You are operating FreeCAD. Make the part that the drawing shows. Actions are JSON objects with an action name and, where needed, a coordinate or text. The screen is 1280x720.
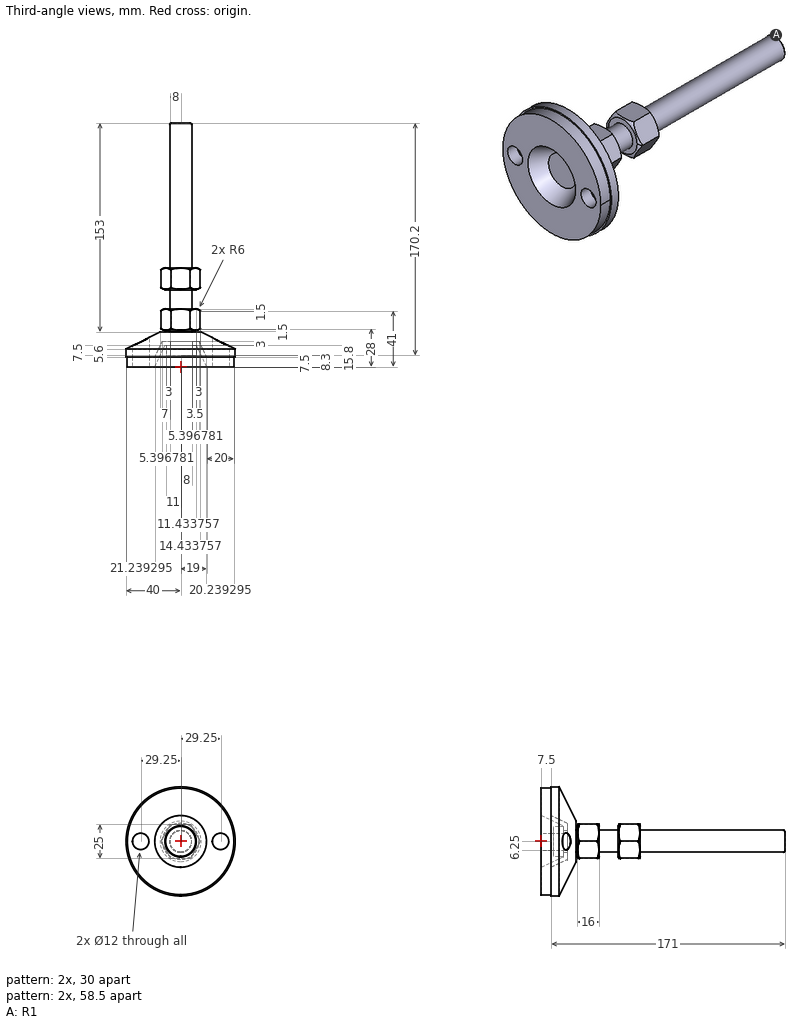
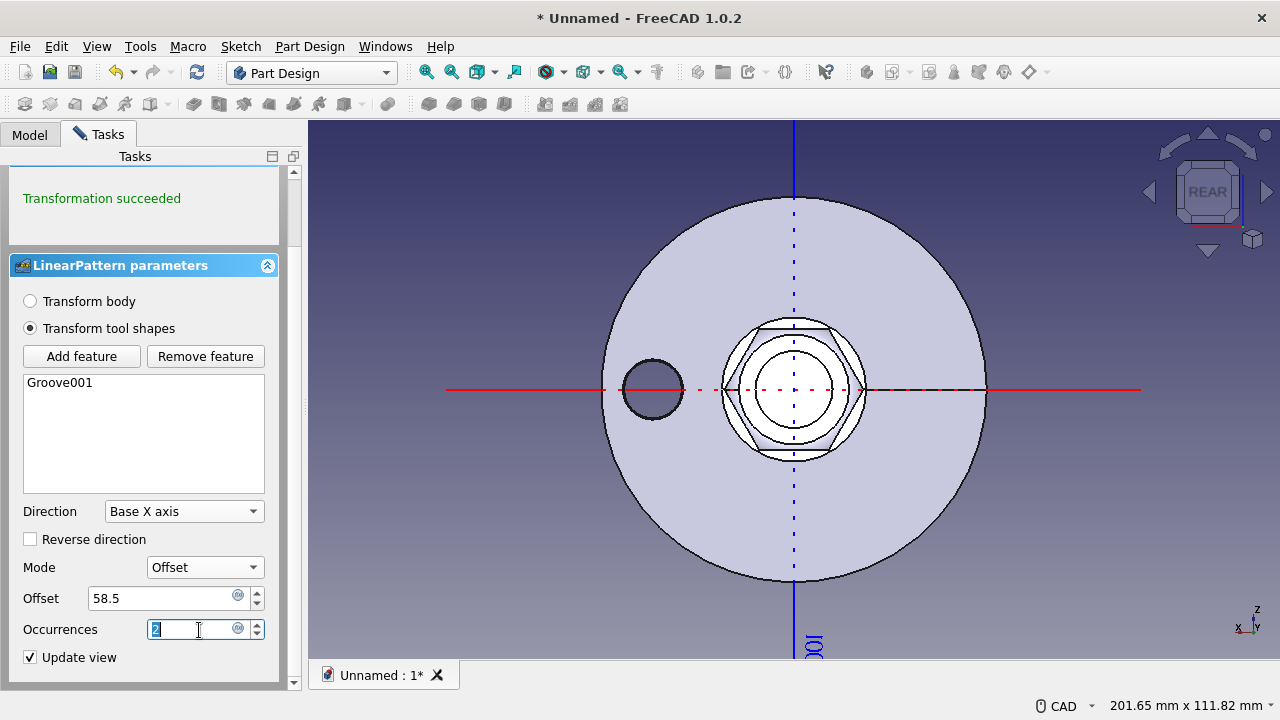
{"action": "type", "text": "2"}
{"action": "key", "text": "Tab"}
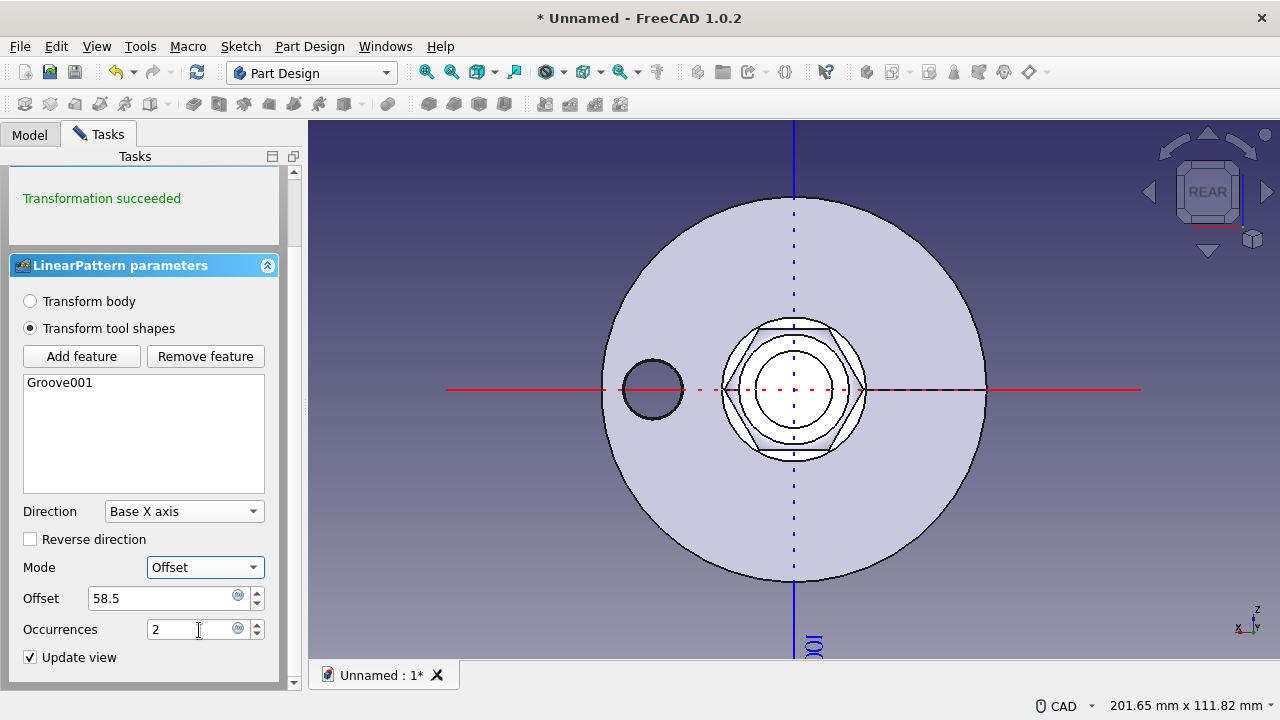
{"action": "left_click", "coordinate": [31, 539]}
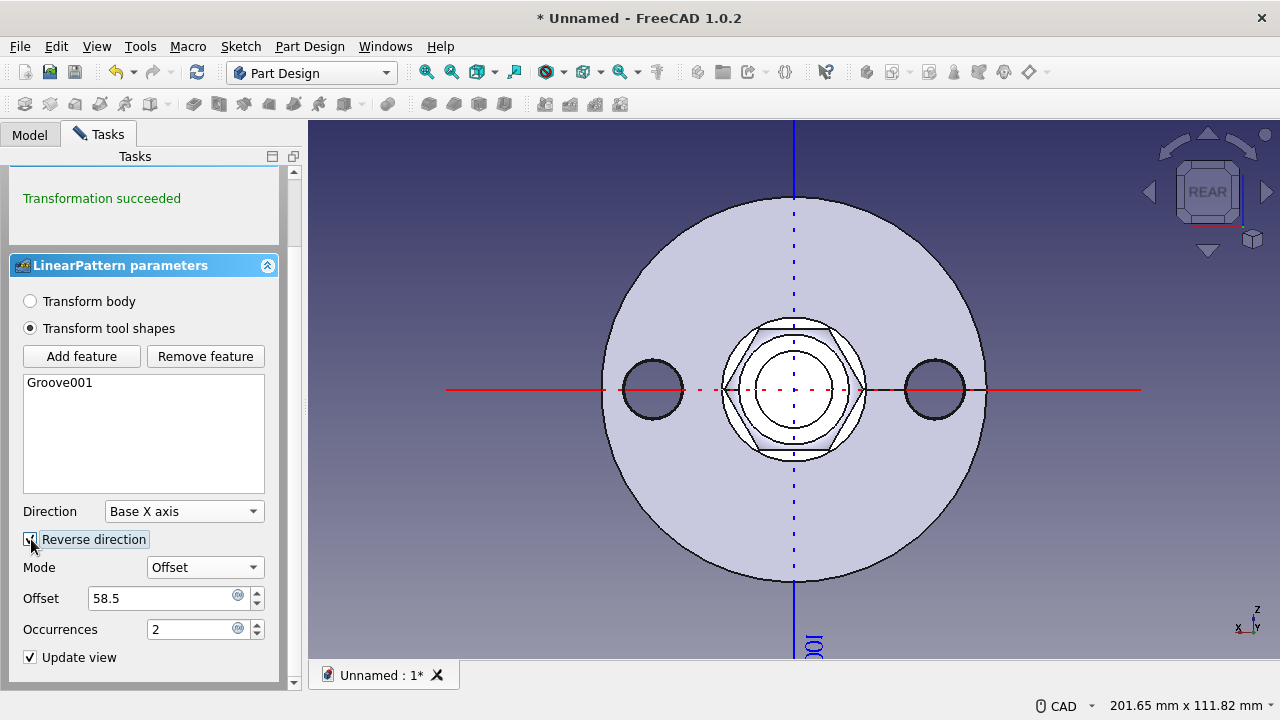
{"action": "scroll", "coordinate": [294, 428], "scroll_direction": "up", "scroll_amount": 3}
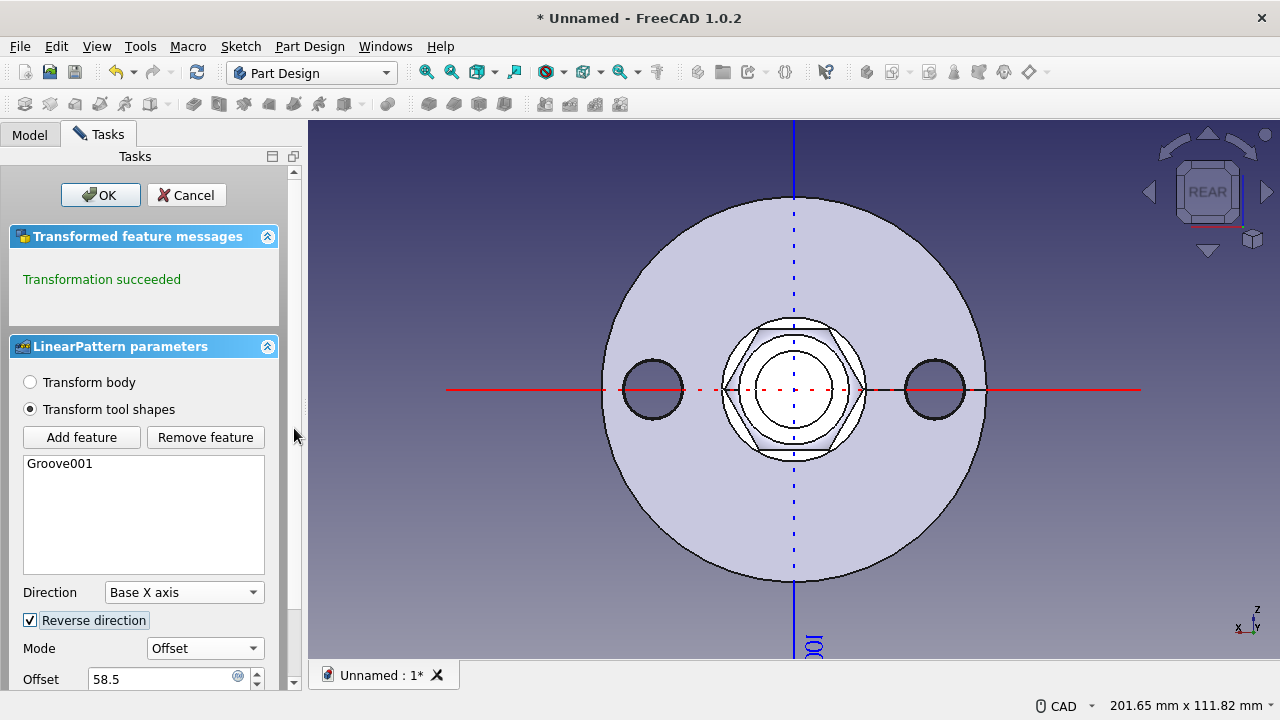
{"action": "left_click", "coordinate": [101, 195]}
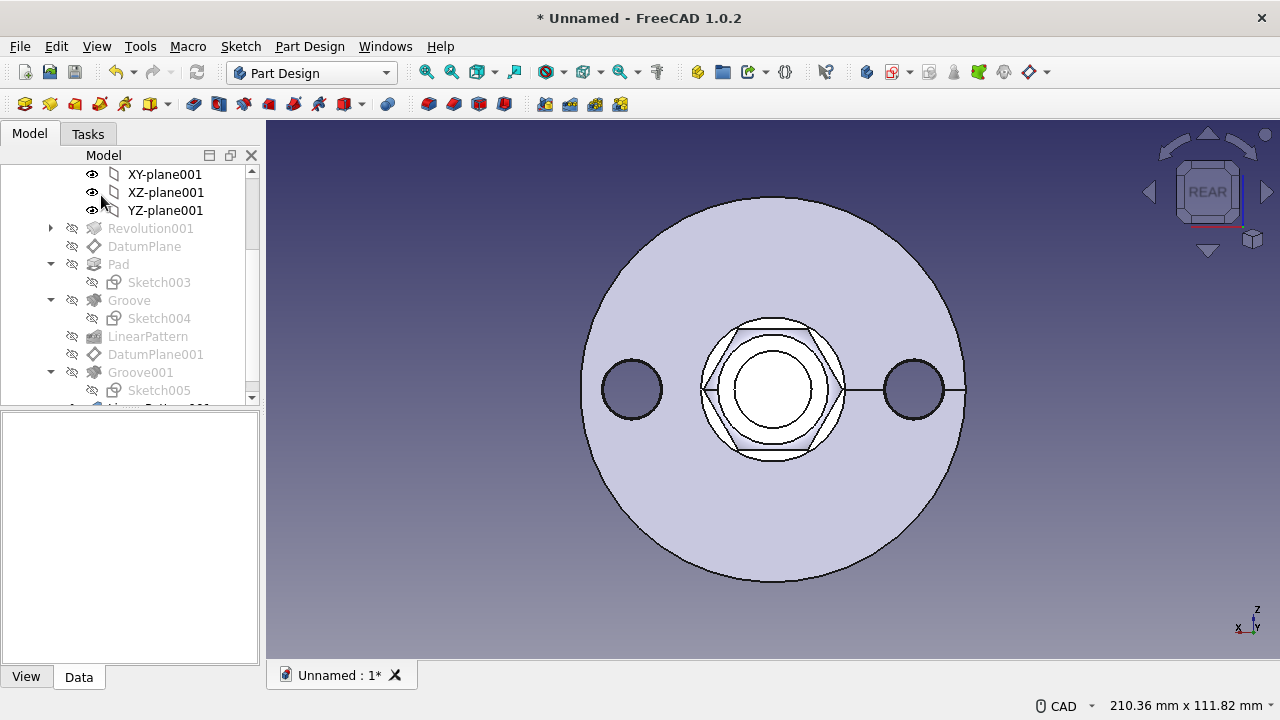
{"action": "left_click", "coordinate": [742, 366]}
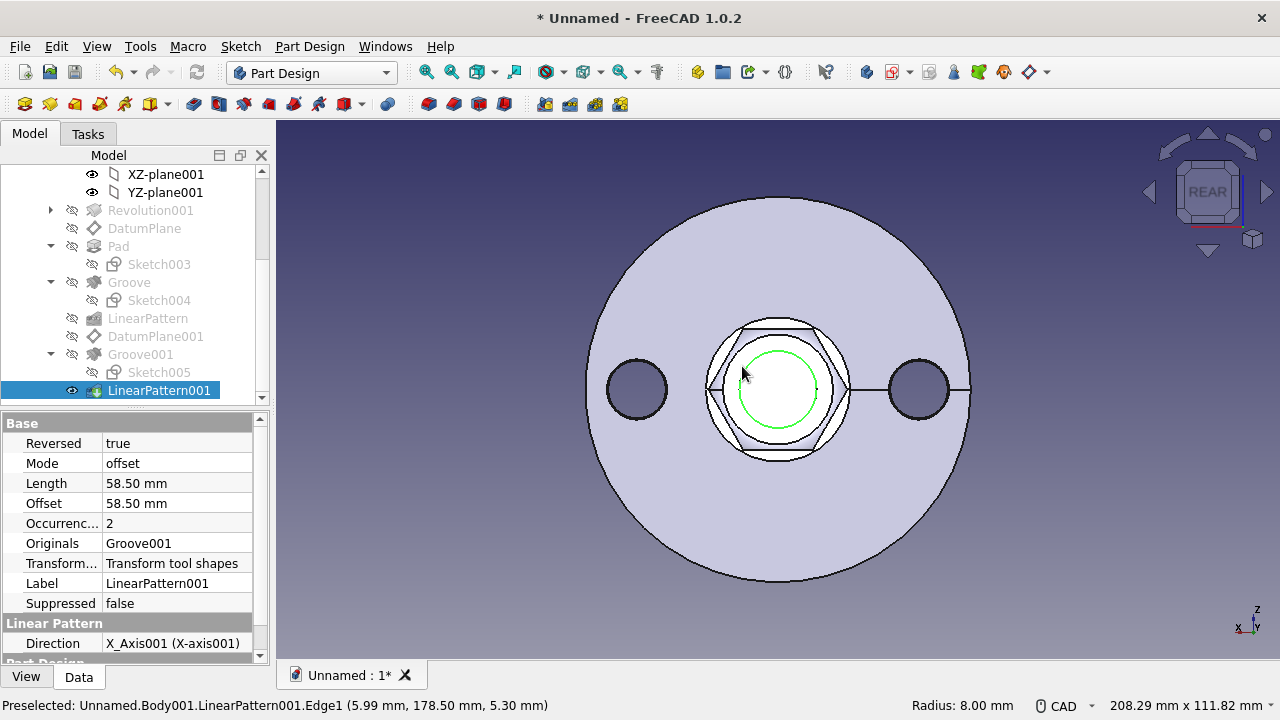
{"action": "left_click", "coordinate": [429, 104]}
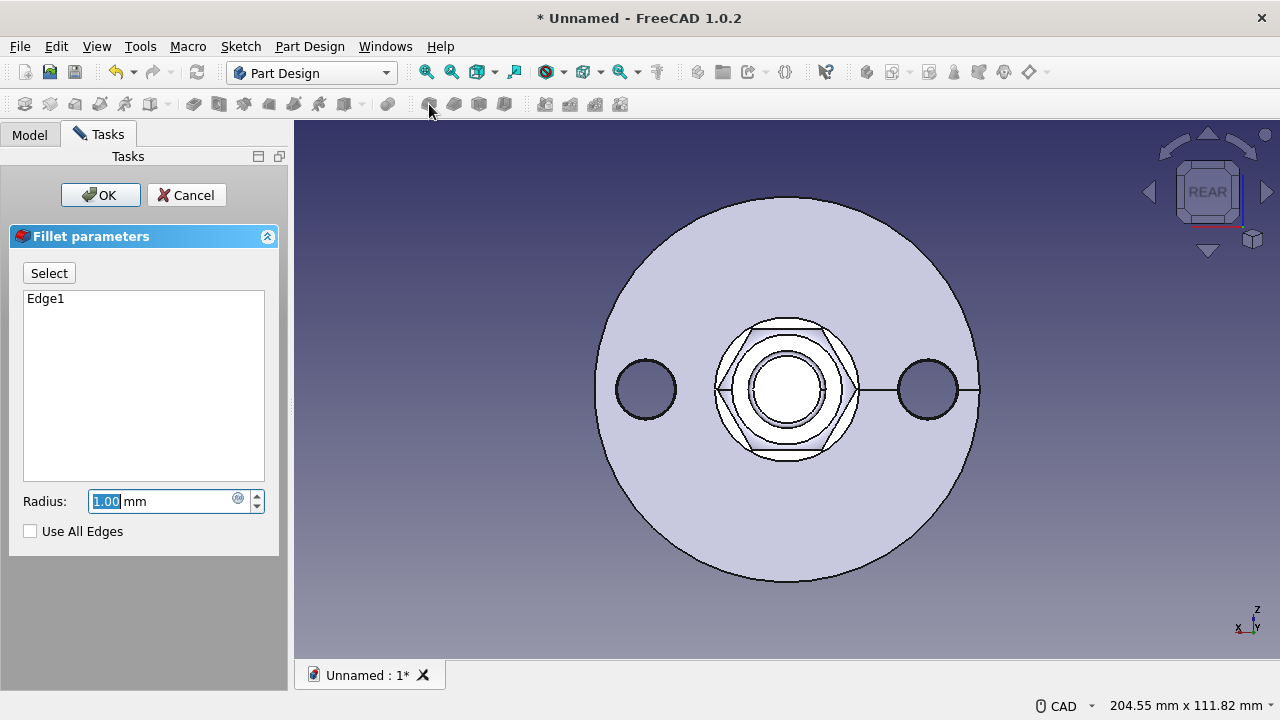
{"action": "type", "text": "1"}
{"action": "key", "text": "Tab"}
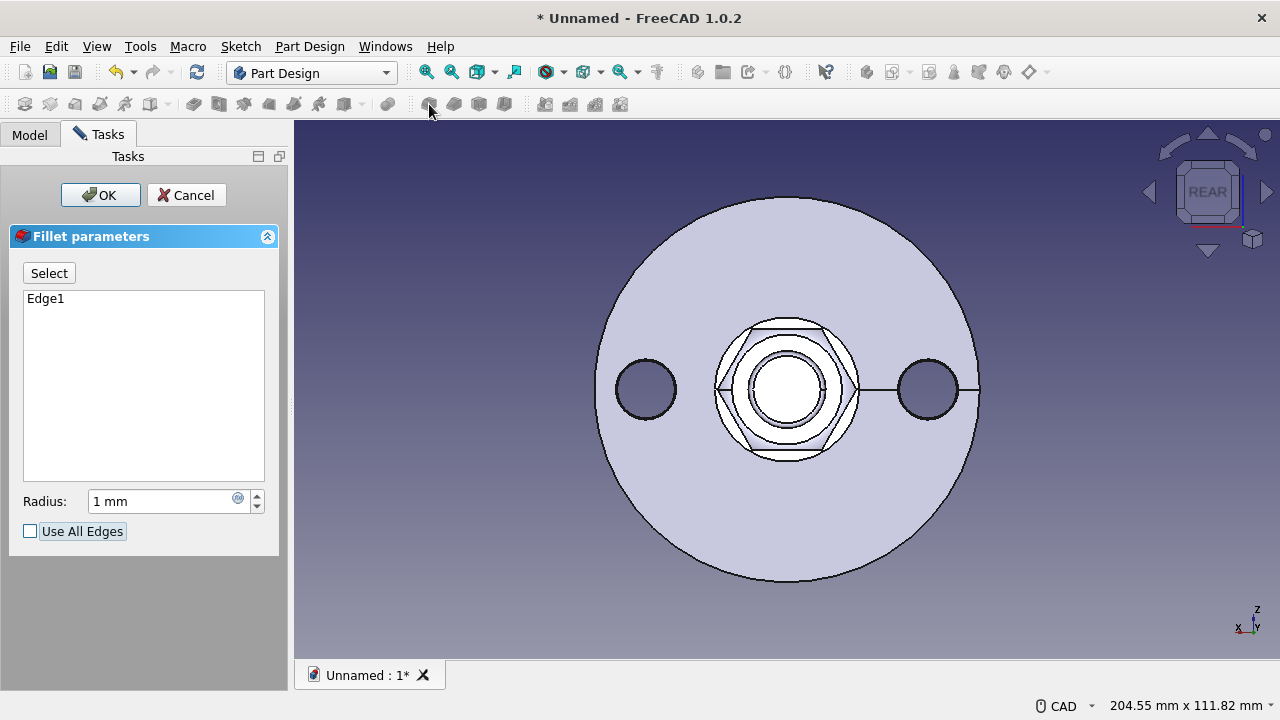
{"action": "left_click", "coordinate": [101, 195]}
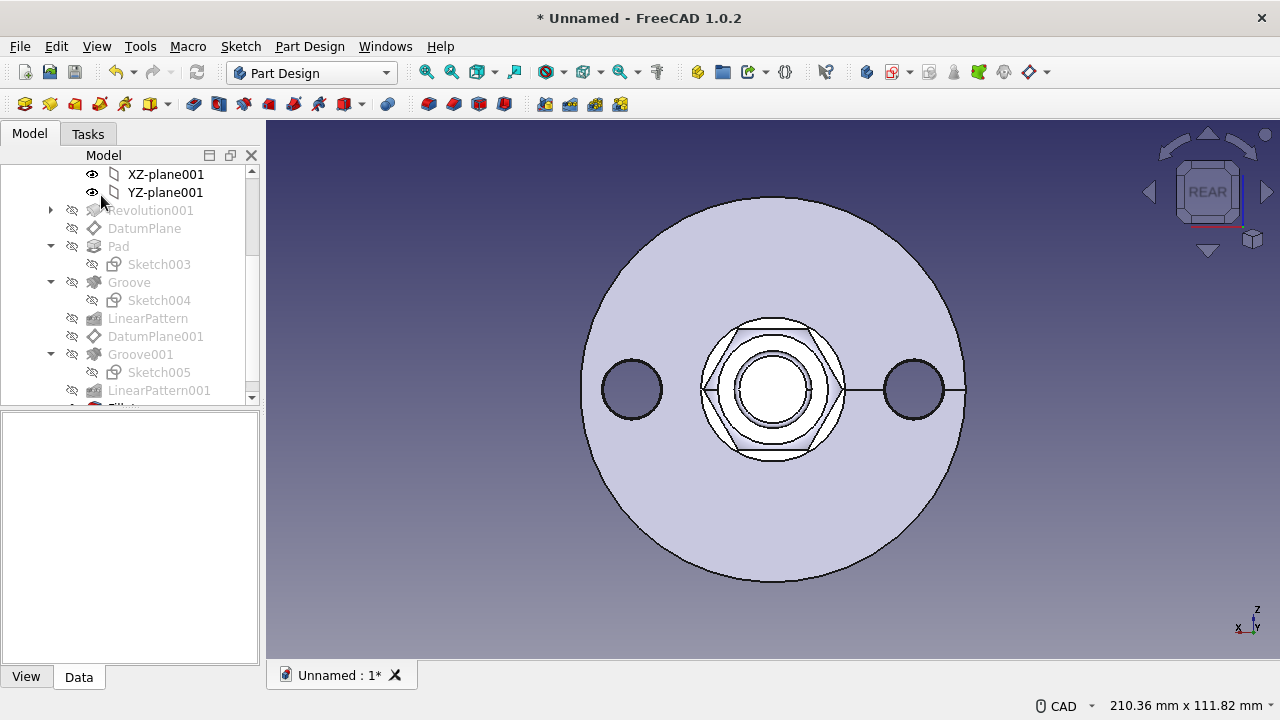
{"action": "key", "text": "0"}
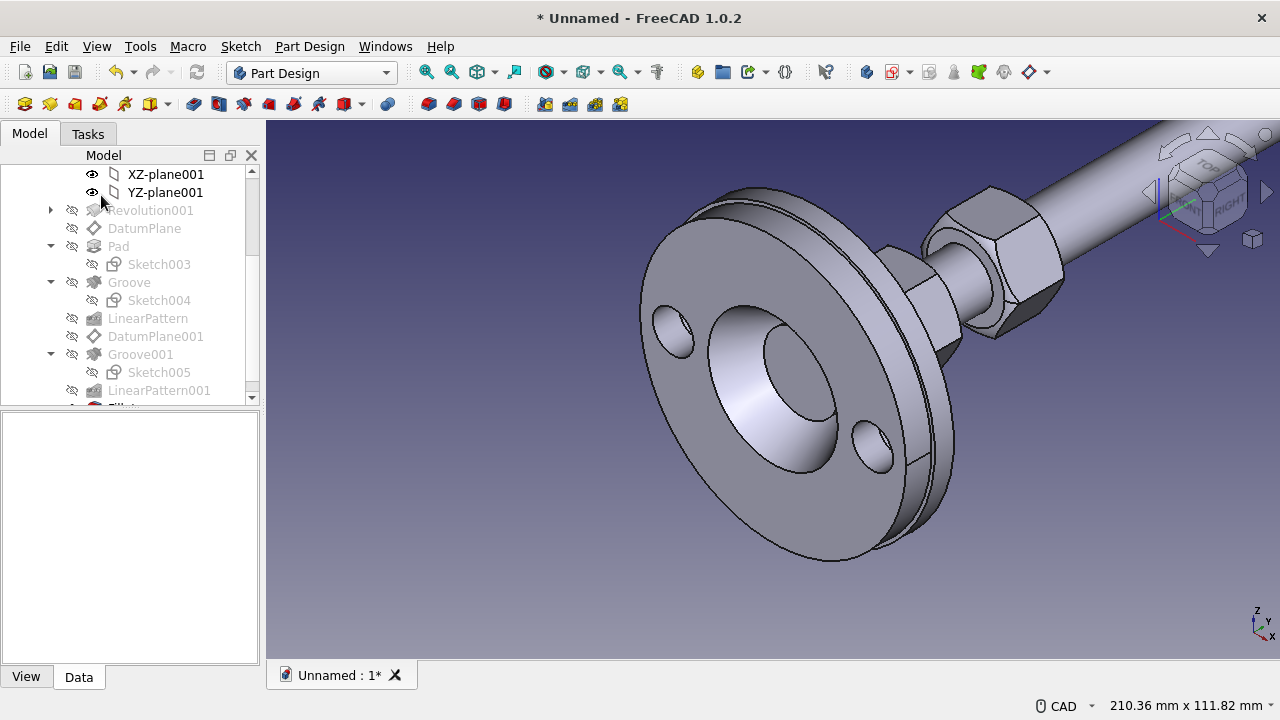
{"action": "left_click", "coordinate": [427, 72]}